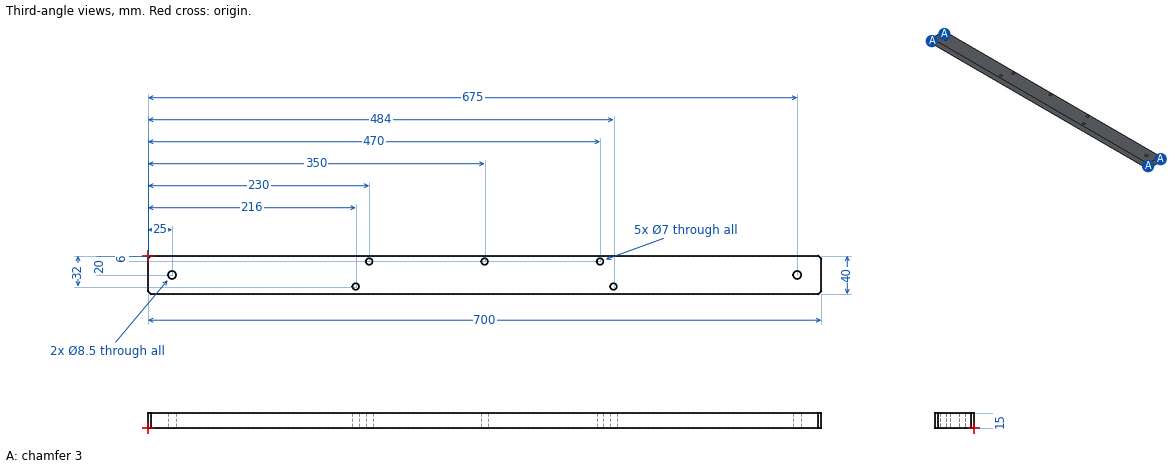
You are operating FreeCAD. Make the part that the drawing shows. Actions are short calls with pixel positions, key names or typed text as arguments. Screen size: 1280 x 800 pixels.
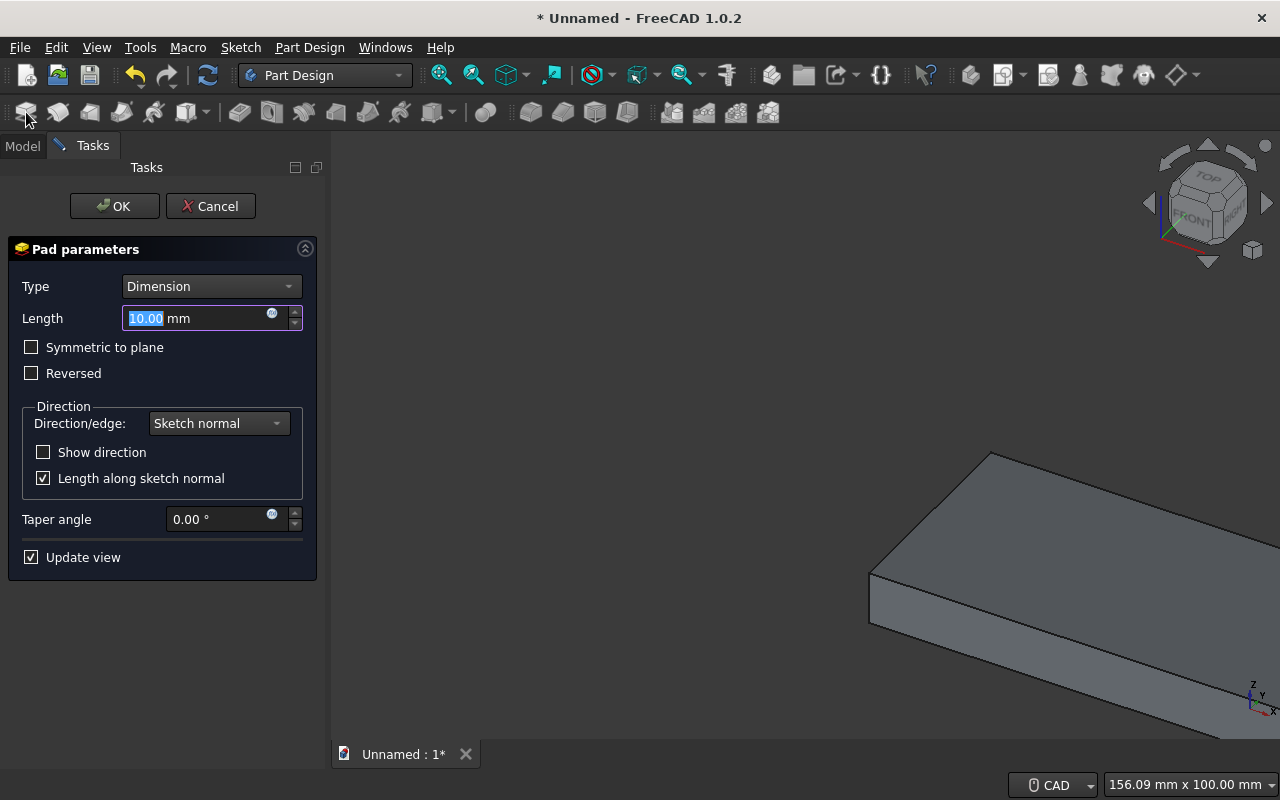
text(15)
key(Tab)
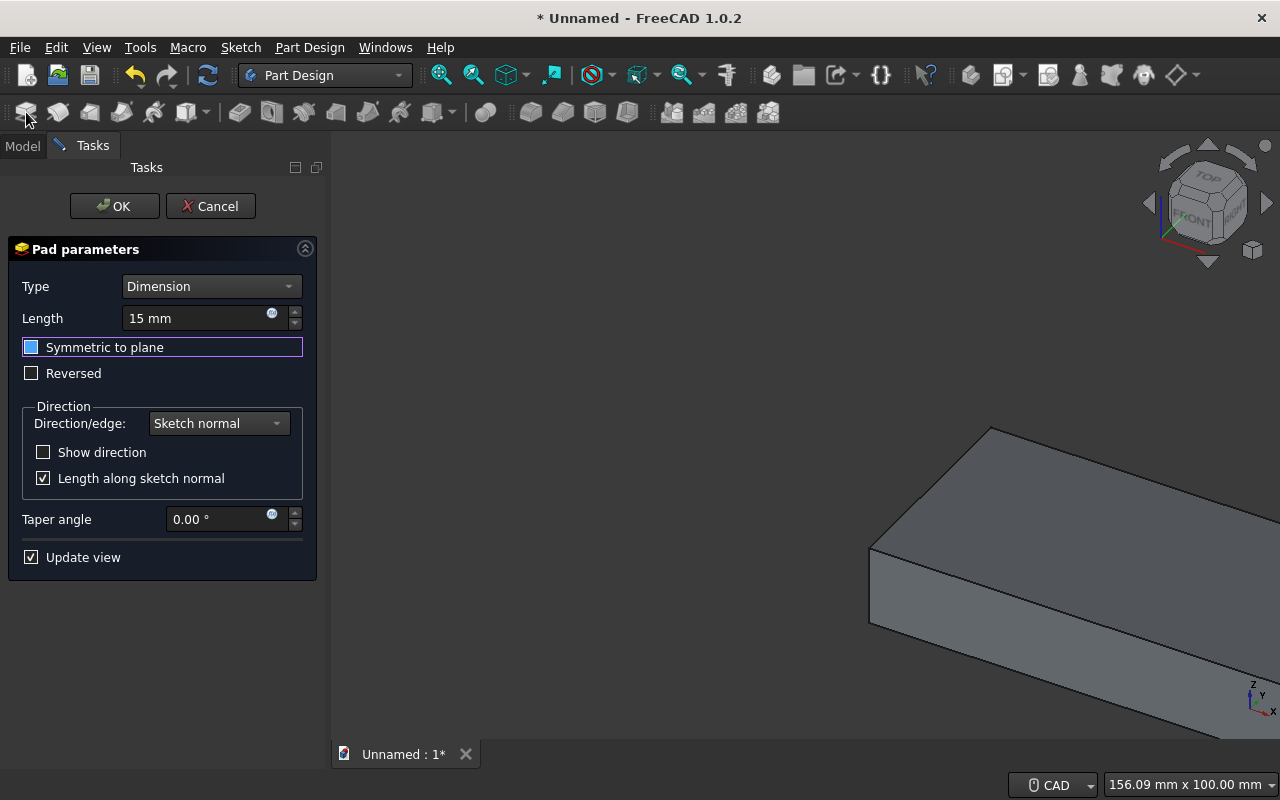
click(115, 206)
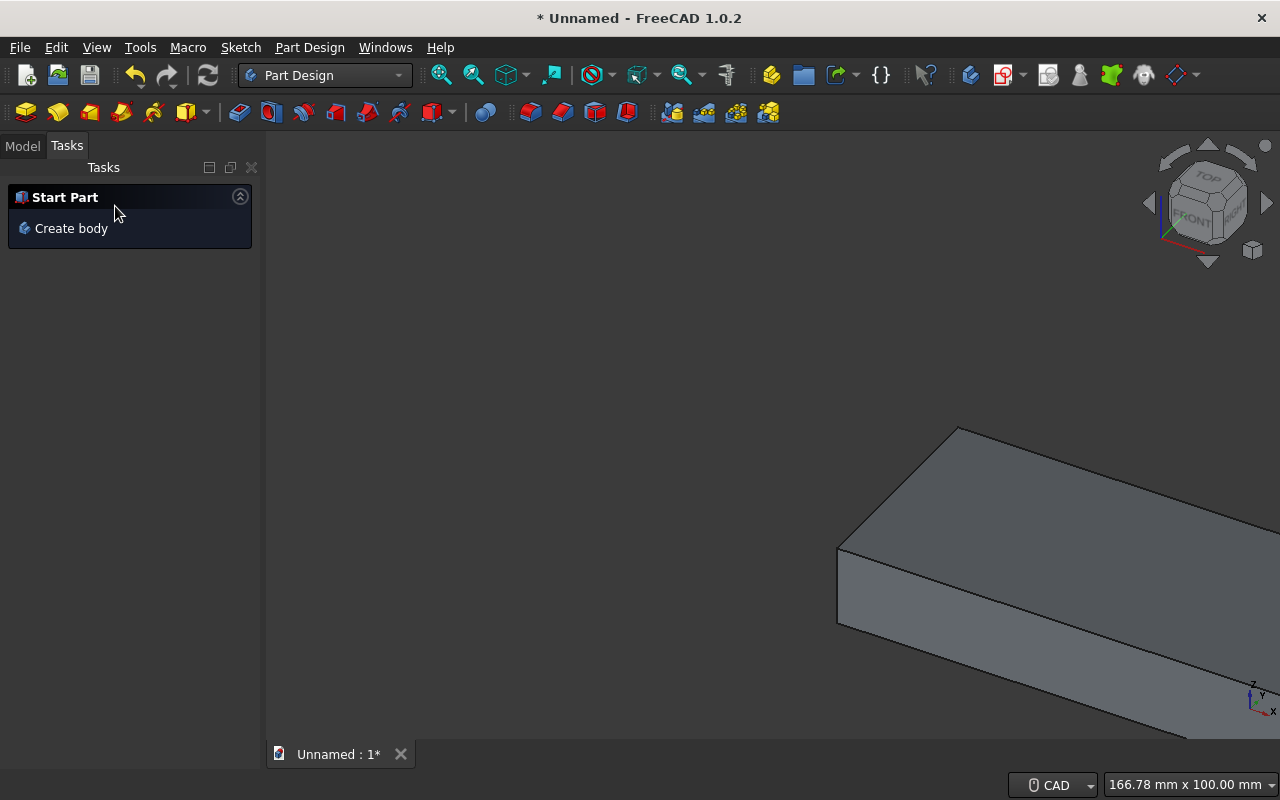
click(442, 76)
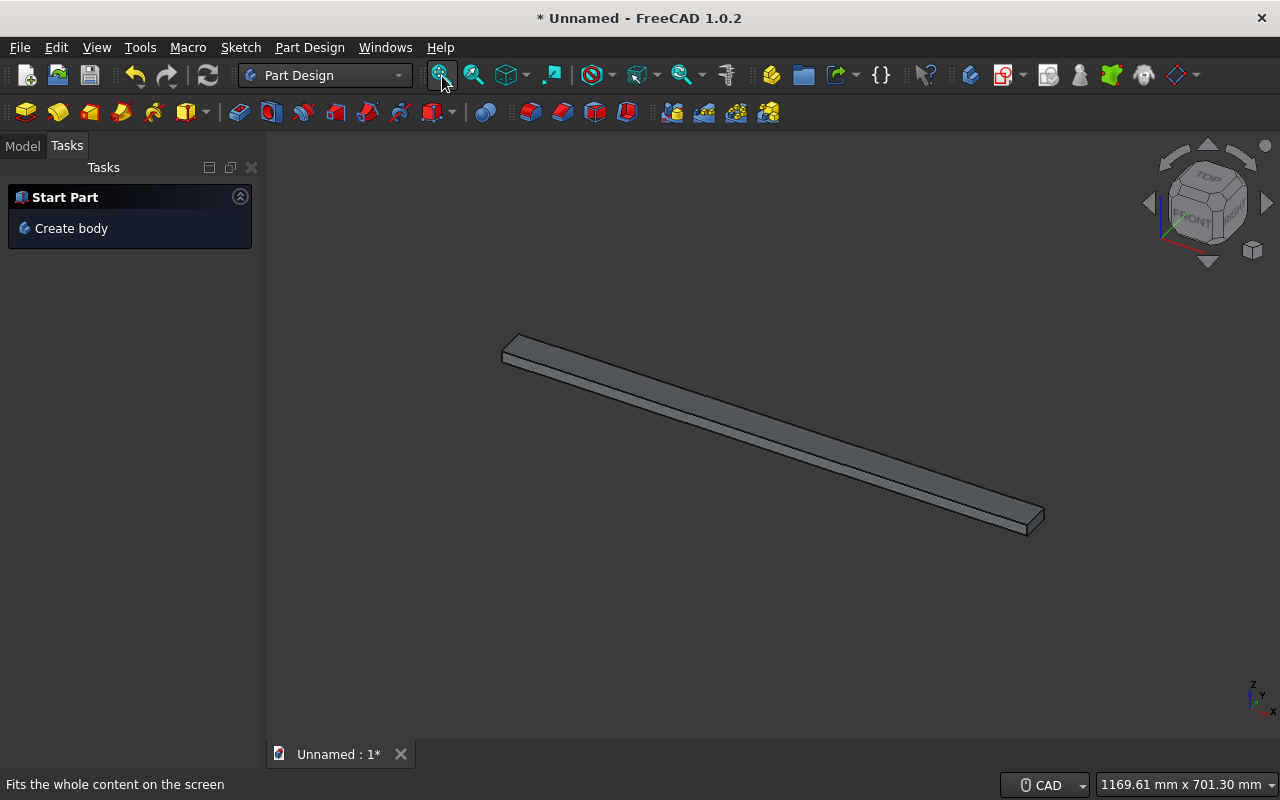
click(1027, 531)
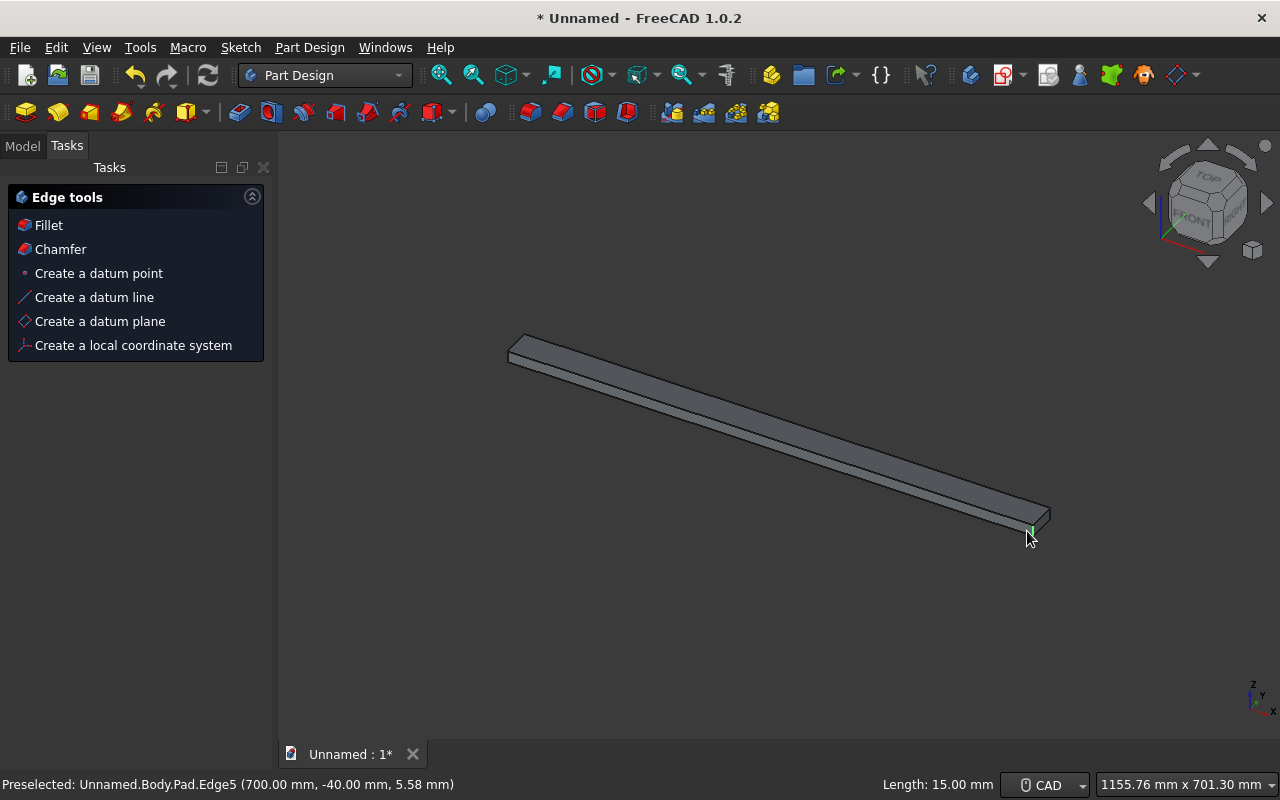
scroll(525, 338, up, 6)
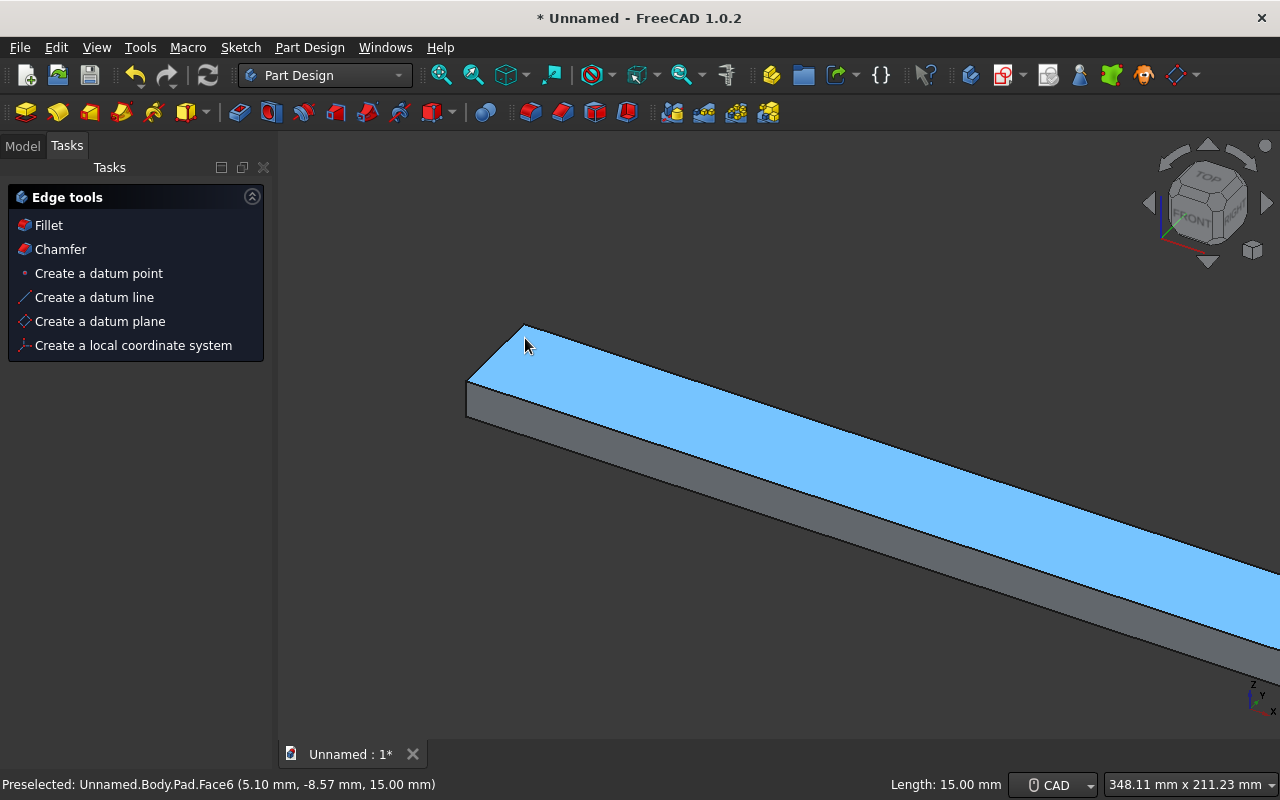
click(442, 76)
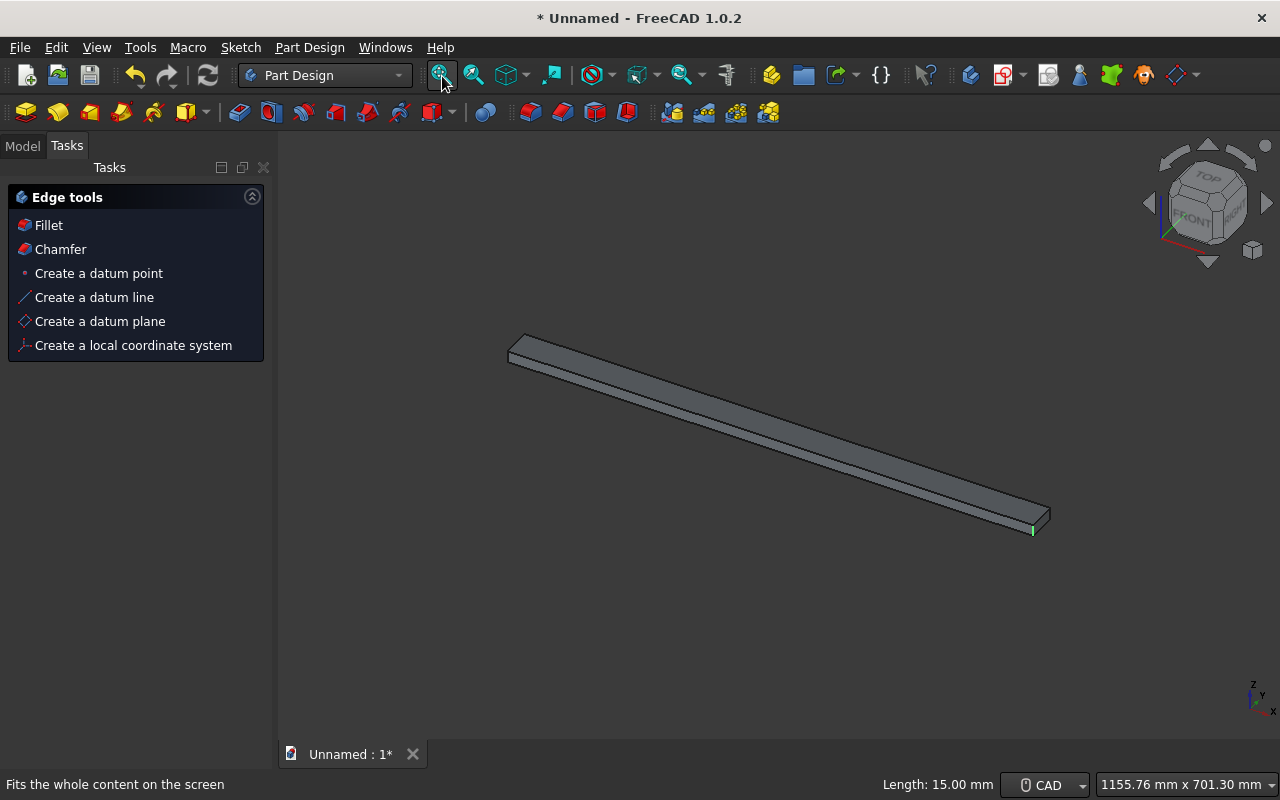
key(0)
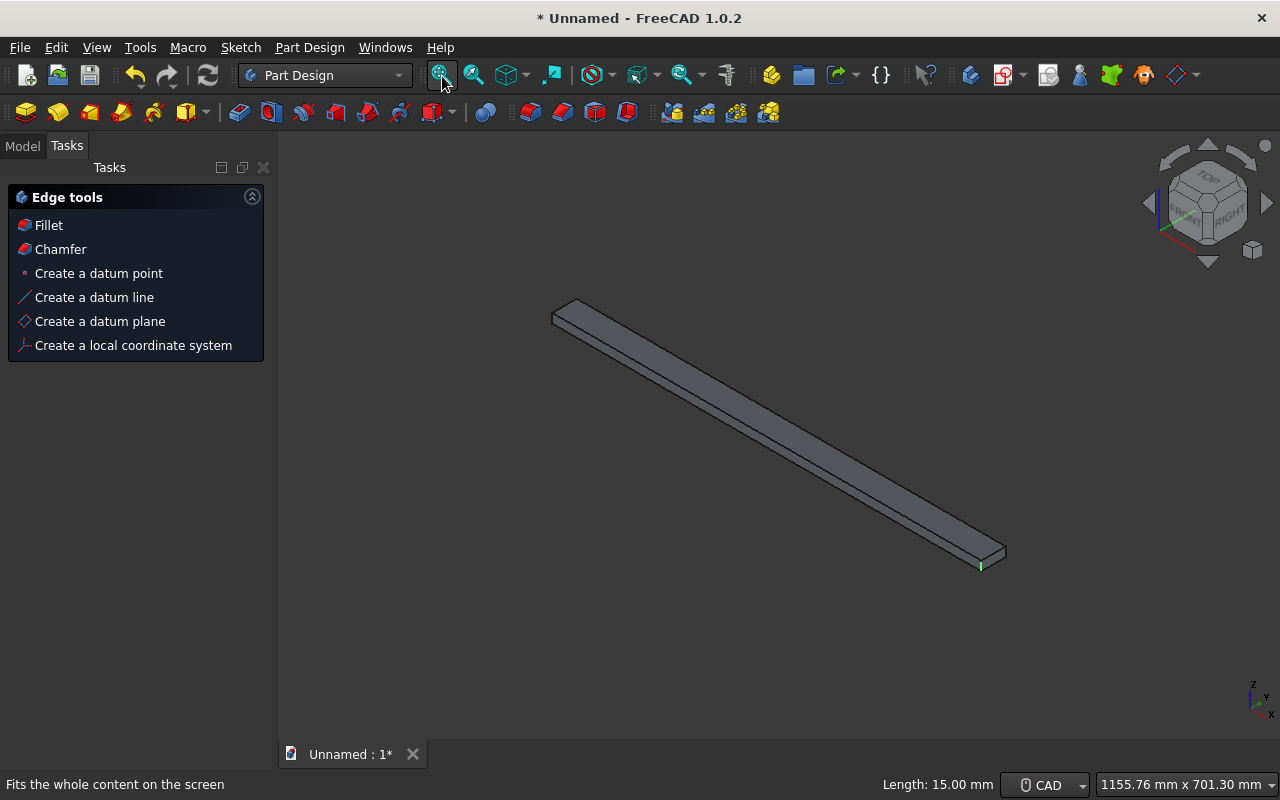
scroll(577, 303, up, 6)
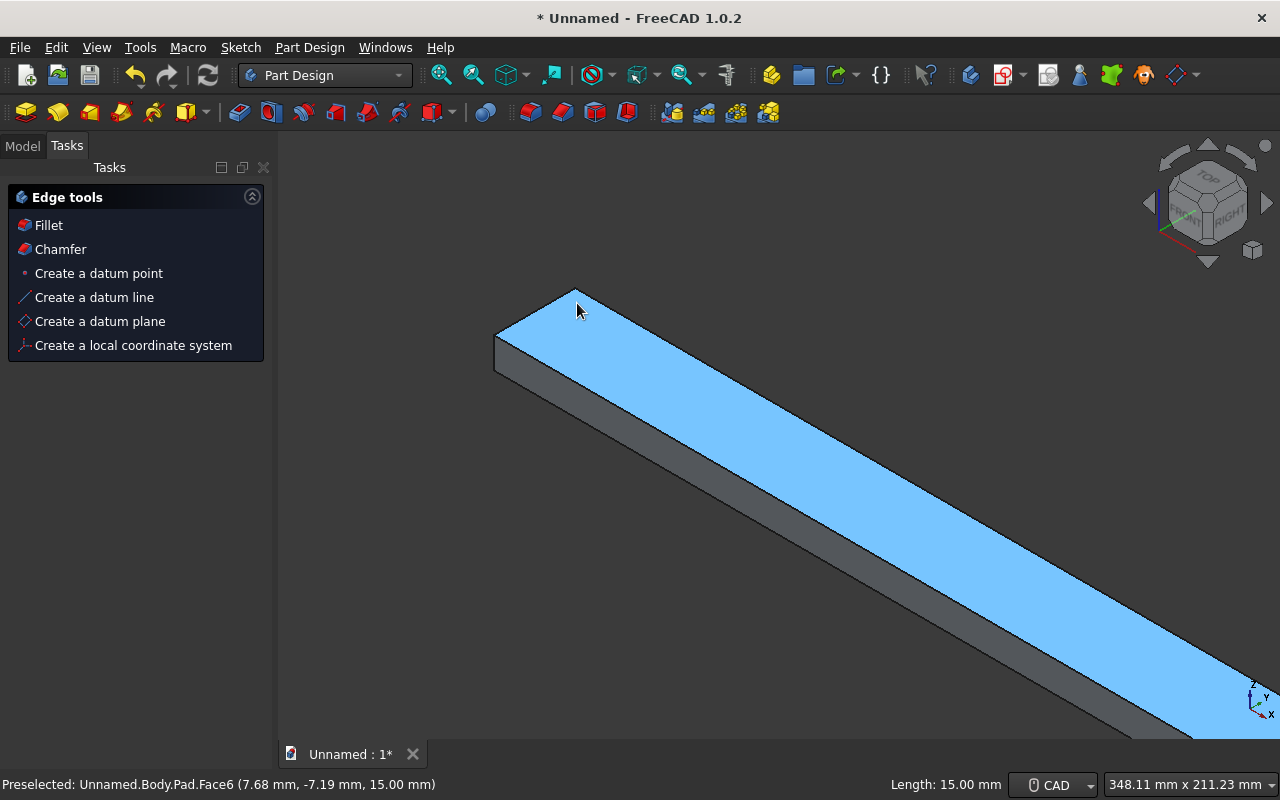
click(442, 76)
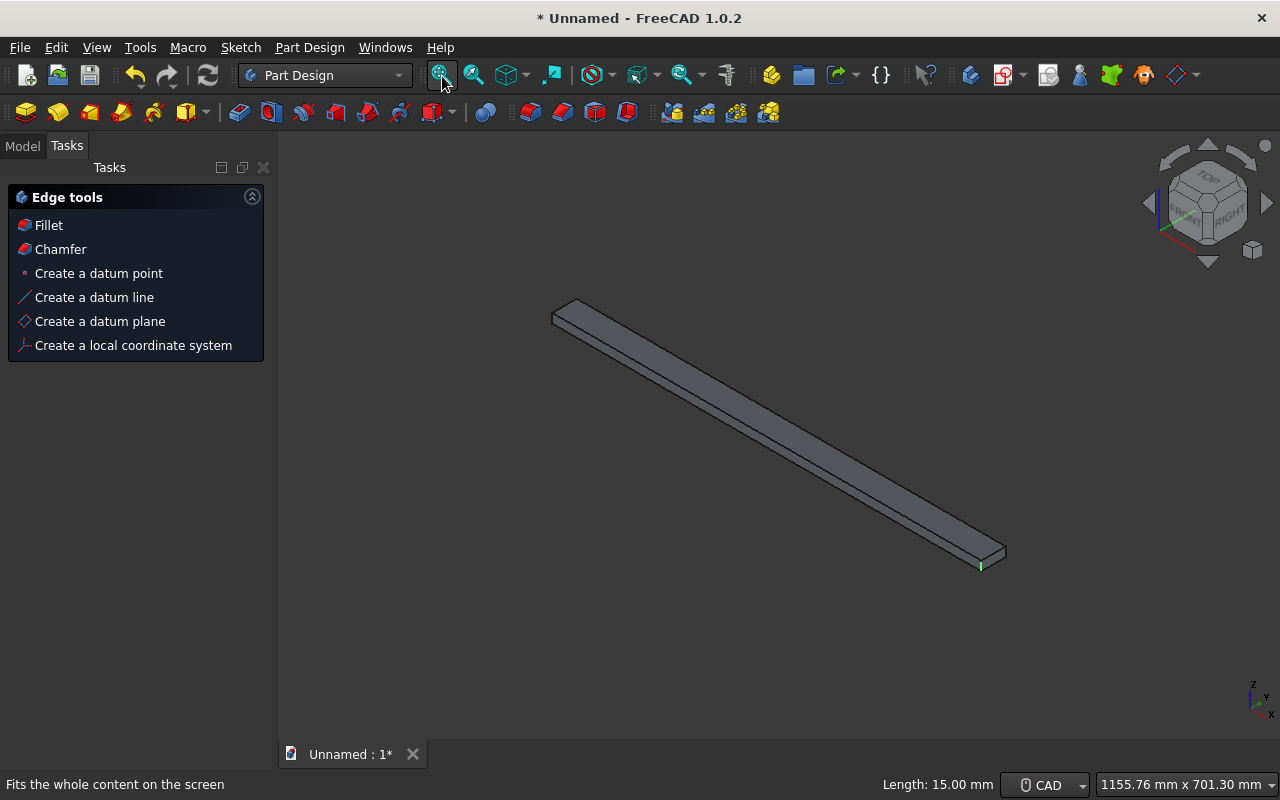
key(2)